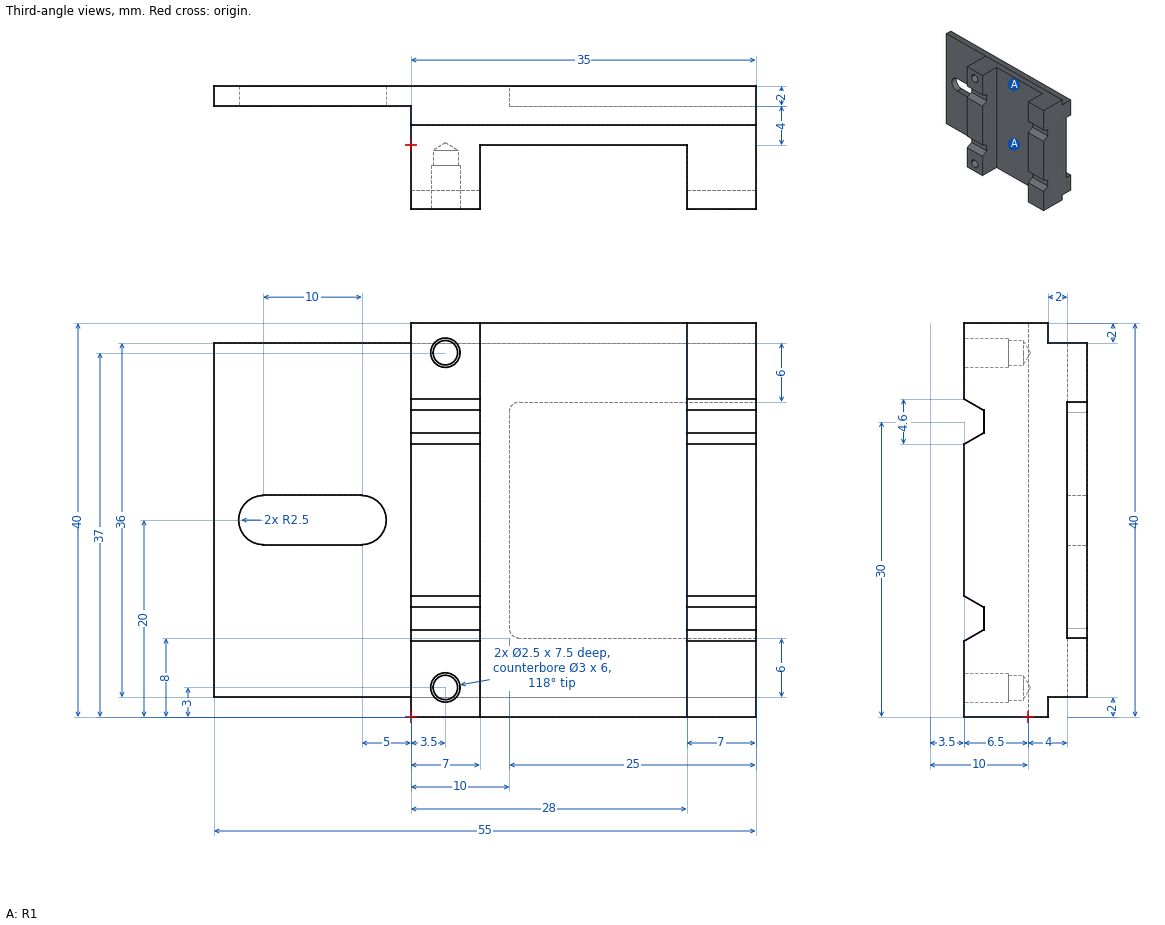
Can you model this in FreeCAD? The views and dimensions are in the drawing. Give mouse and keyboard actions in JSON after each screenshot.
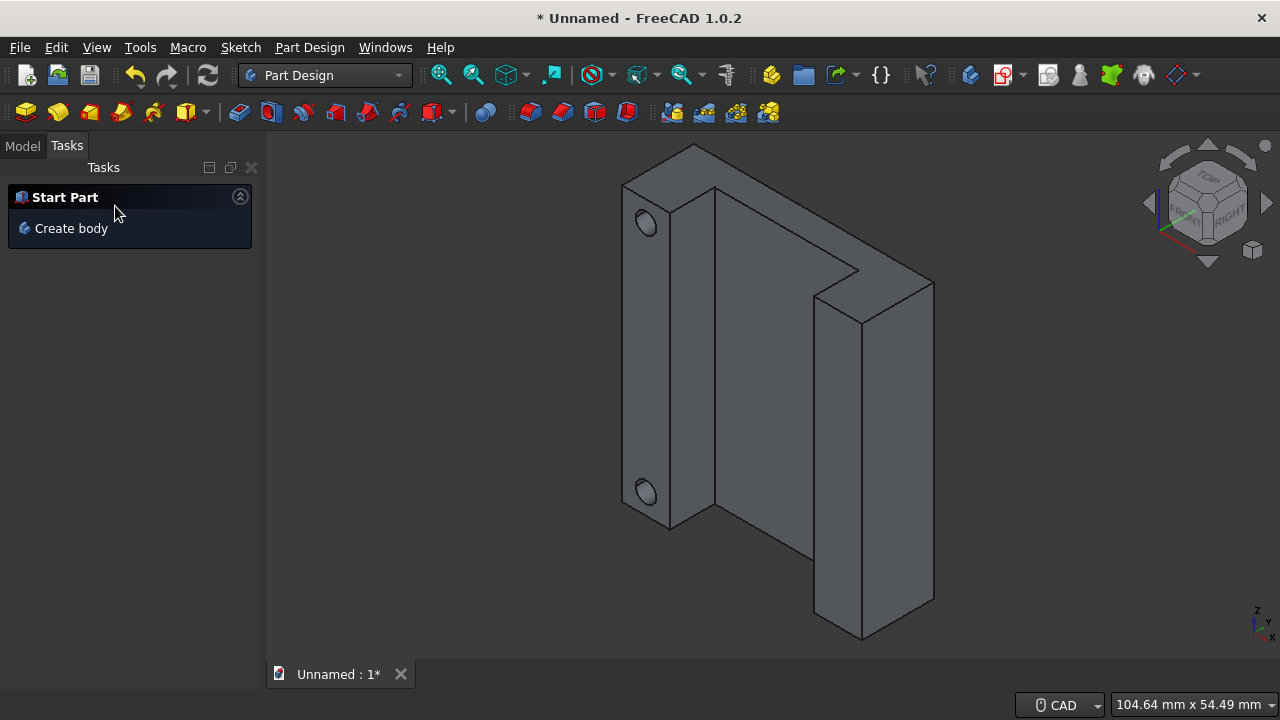
{"action": "key", "text": "6"}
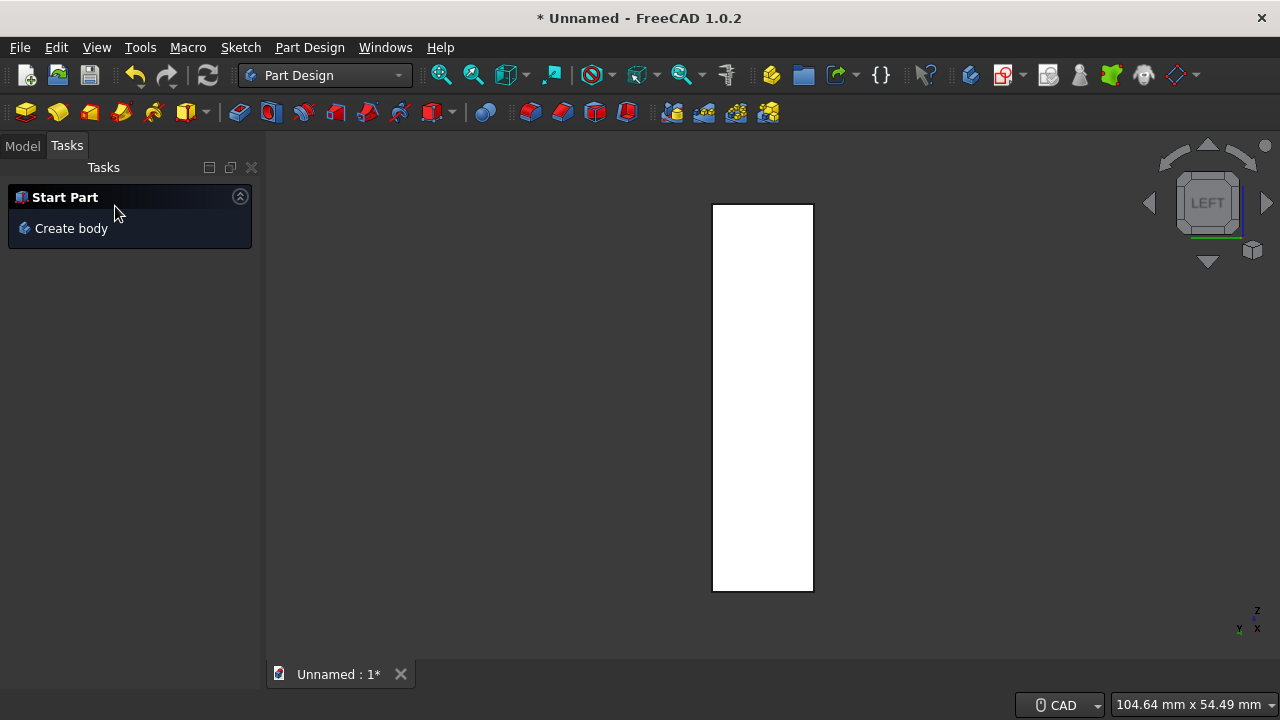
{"action": "left_click", "coordinate": [763, 287]}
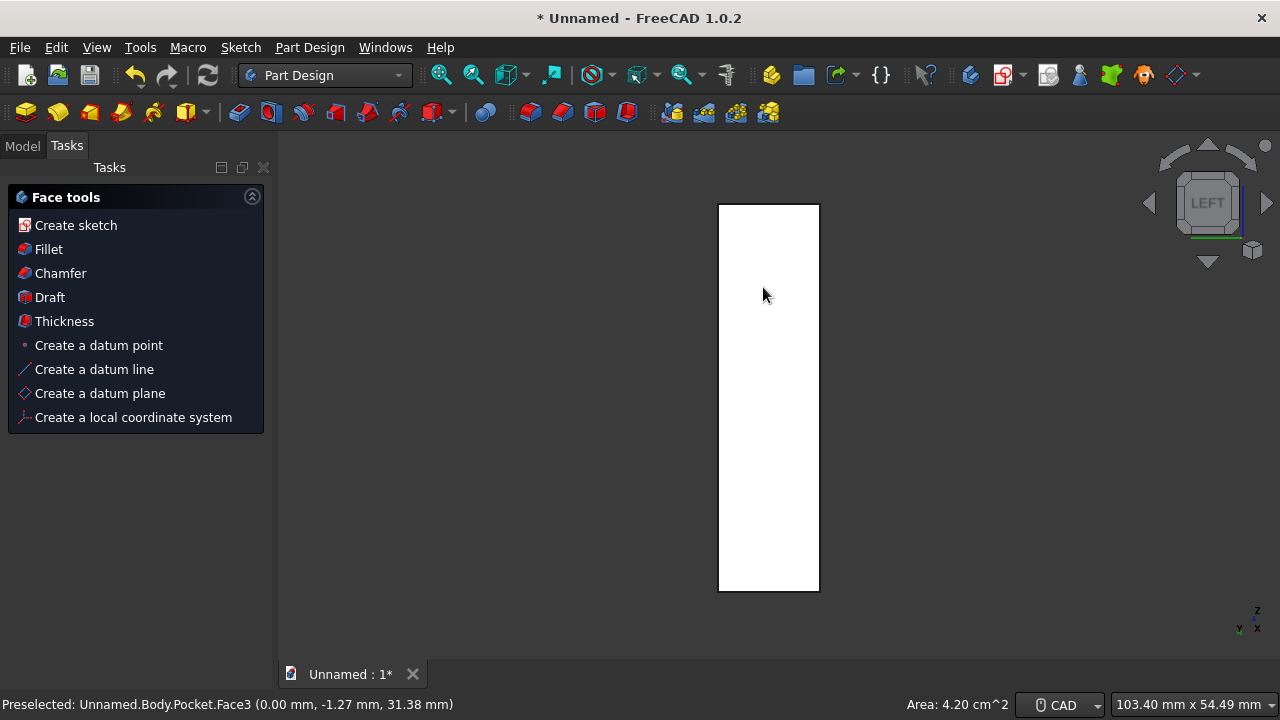
{"action": "left_click", "coordinate": [1004, 76]}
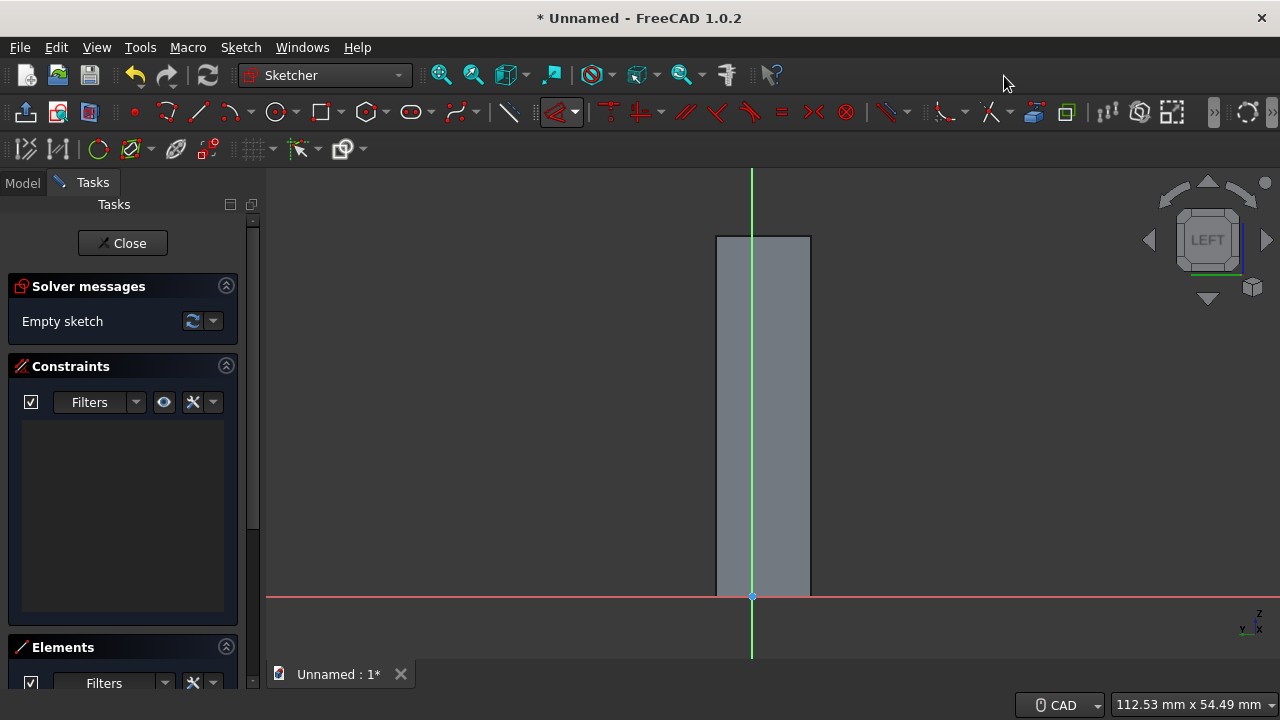
{"action": "left_click", "coordinate": [322, 112]}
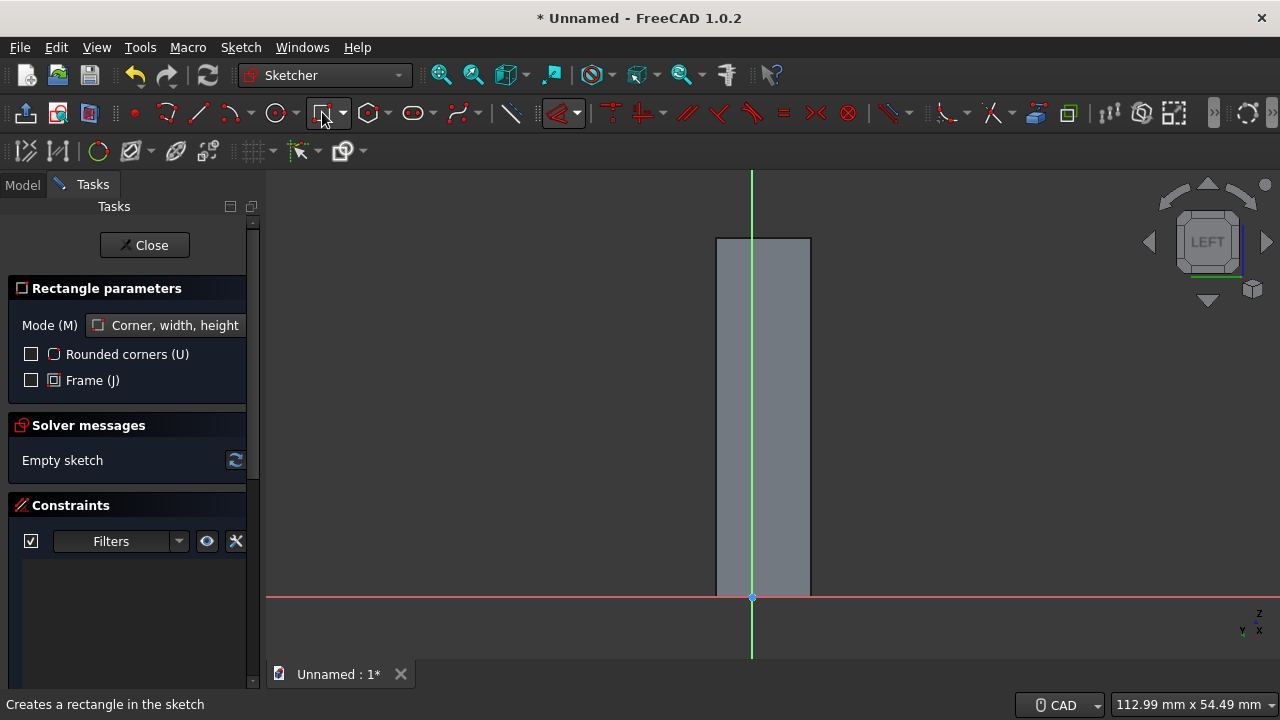
{"action": "left_click", "coordinate": [716, 579]}
{"action": "left_click", "coordinate": [734, 597]}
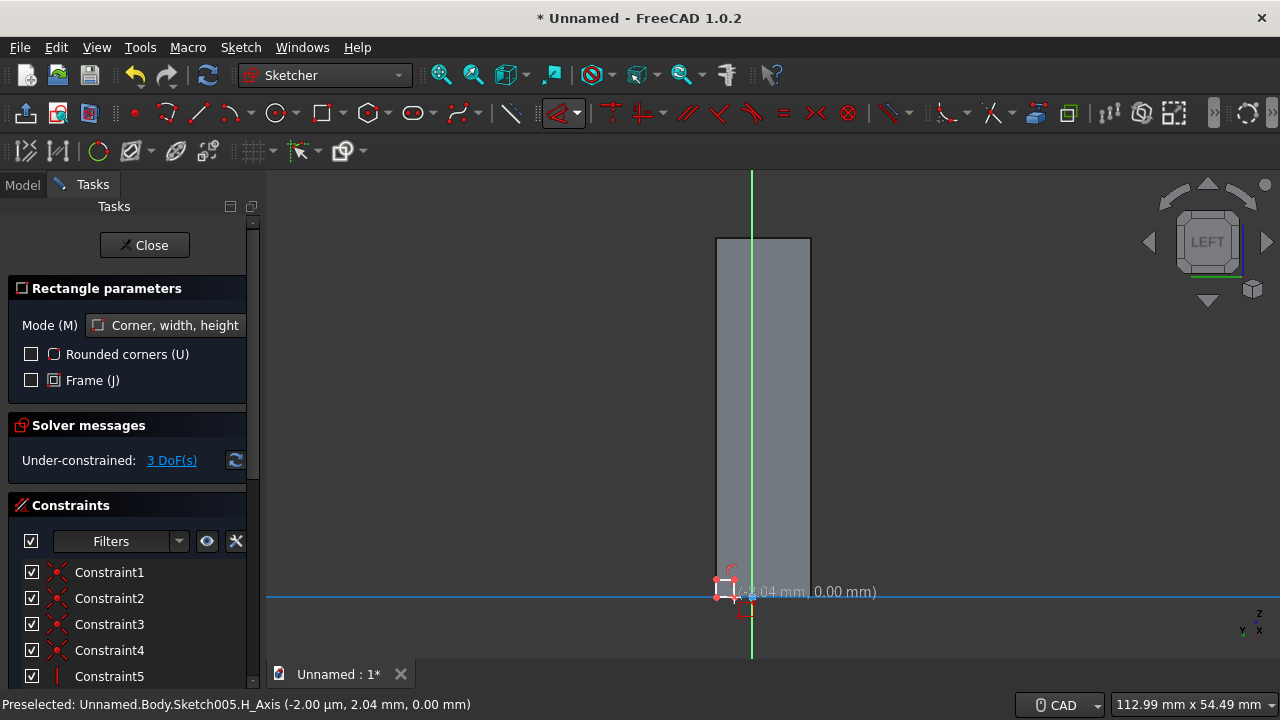
{"action": "left_click", "coordinate": [716, 238]}
{"action": "mouse_move", "coordinate": [734, 256]}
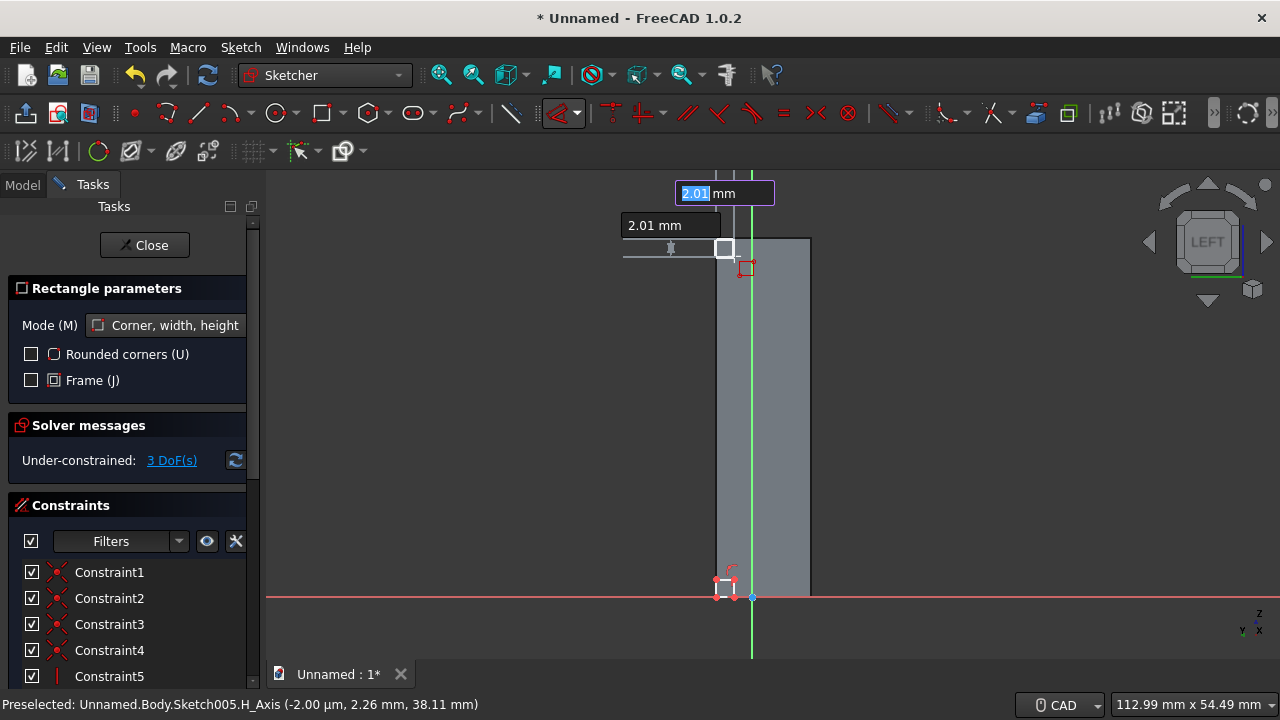
{"action": "type", "text": "2"}
{"action": "key", "text": "Tab"}
{"action": "type", "text": "2"}
{"action": "key", "text": "Return"}
{"action": "key", "text": "Escape"}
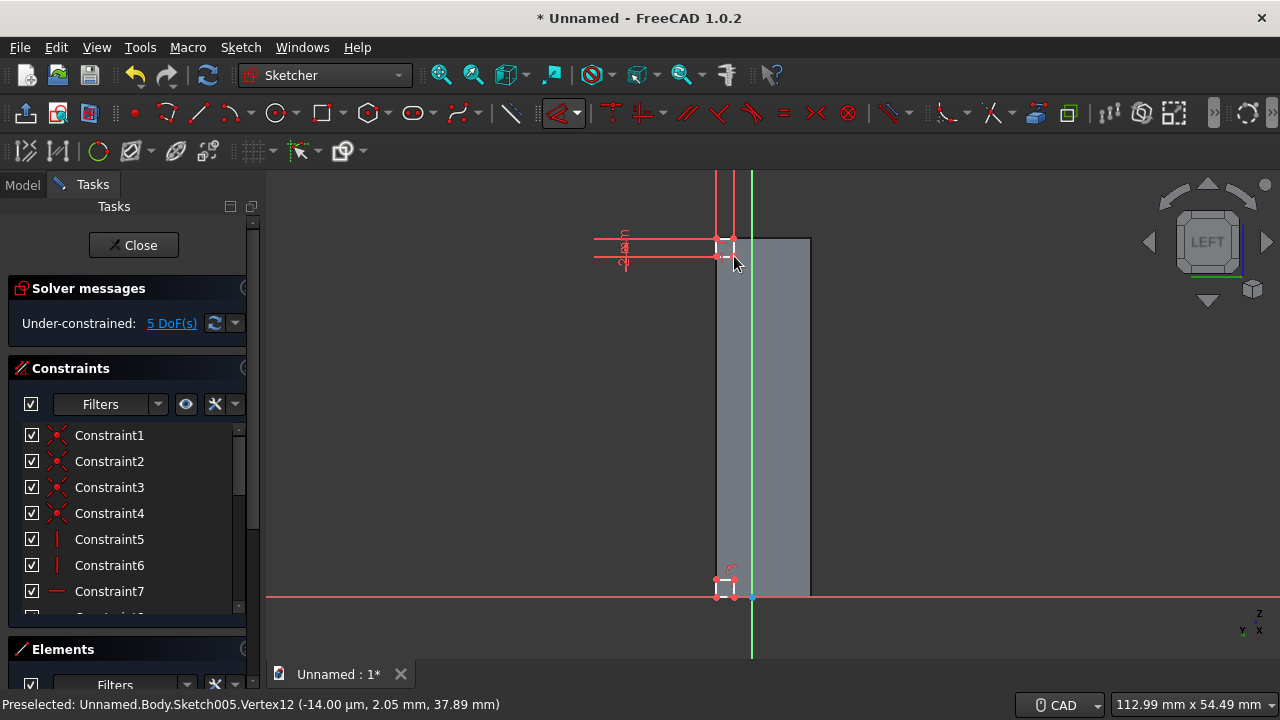
{"action": "scroll", "coordinate": [716, 589], "scroll_direction": "up", "scroll_amount": 4}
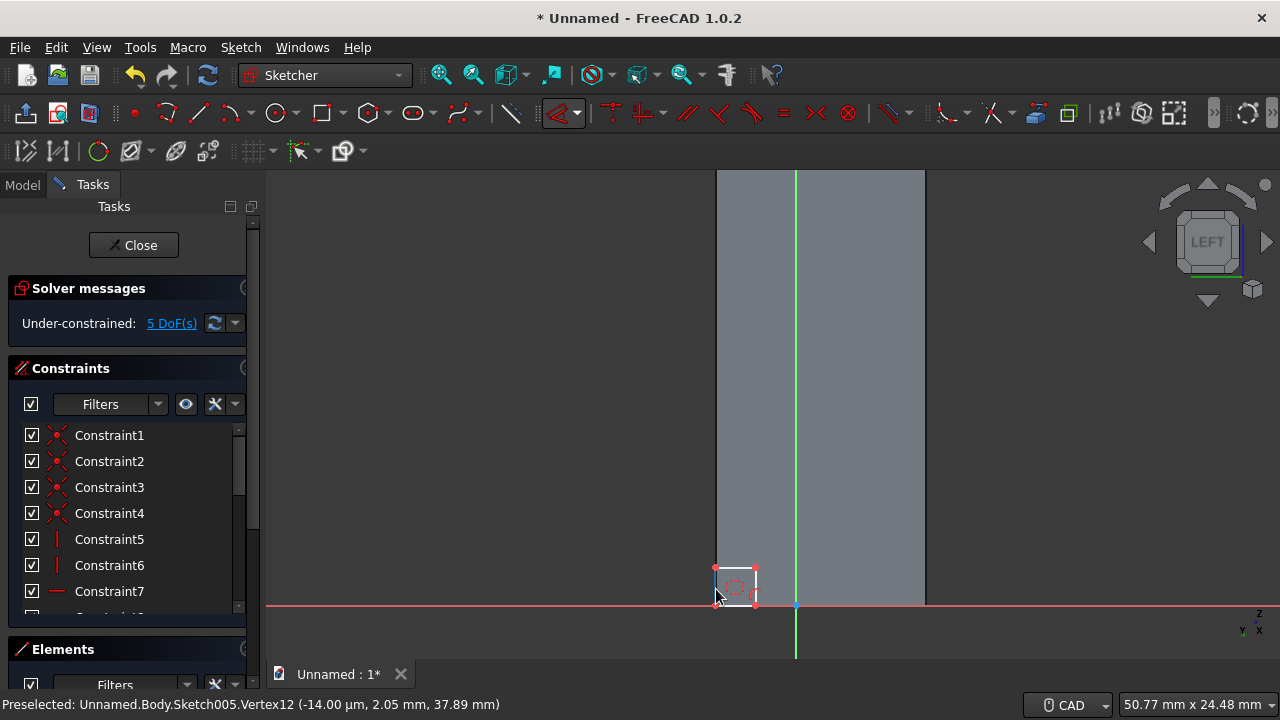
{"action": "left_click", "coordinate": [715, 587]}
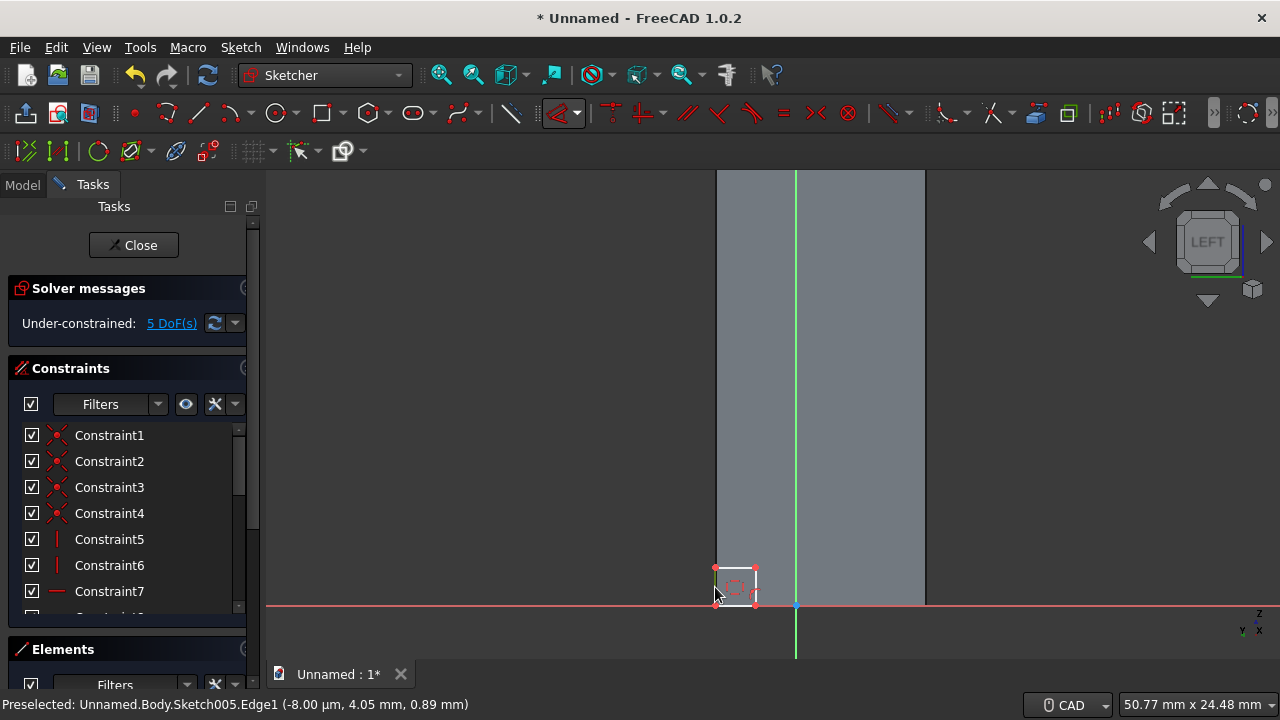
{"action": "left_click", "coordinate": [580, 114]}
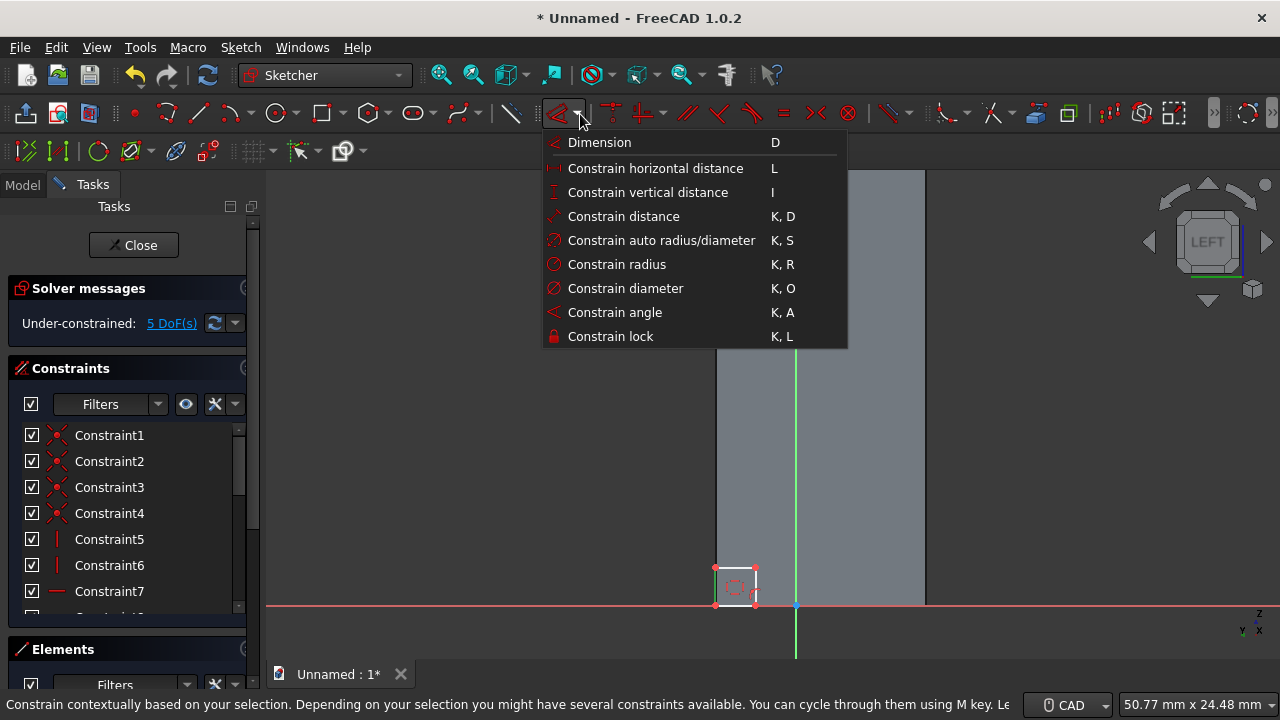
{"action": "left_click", "coordinate": [695, 192]}